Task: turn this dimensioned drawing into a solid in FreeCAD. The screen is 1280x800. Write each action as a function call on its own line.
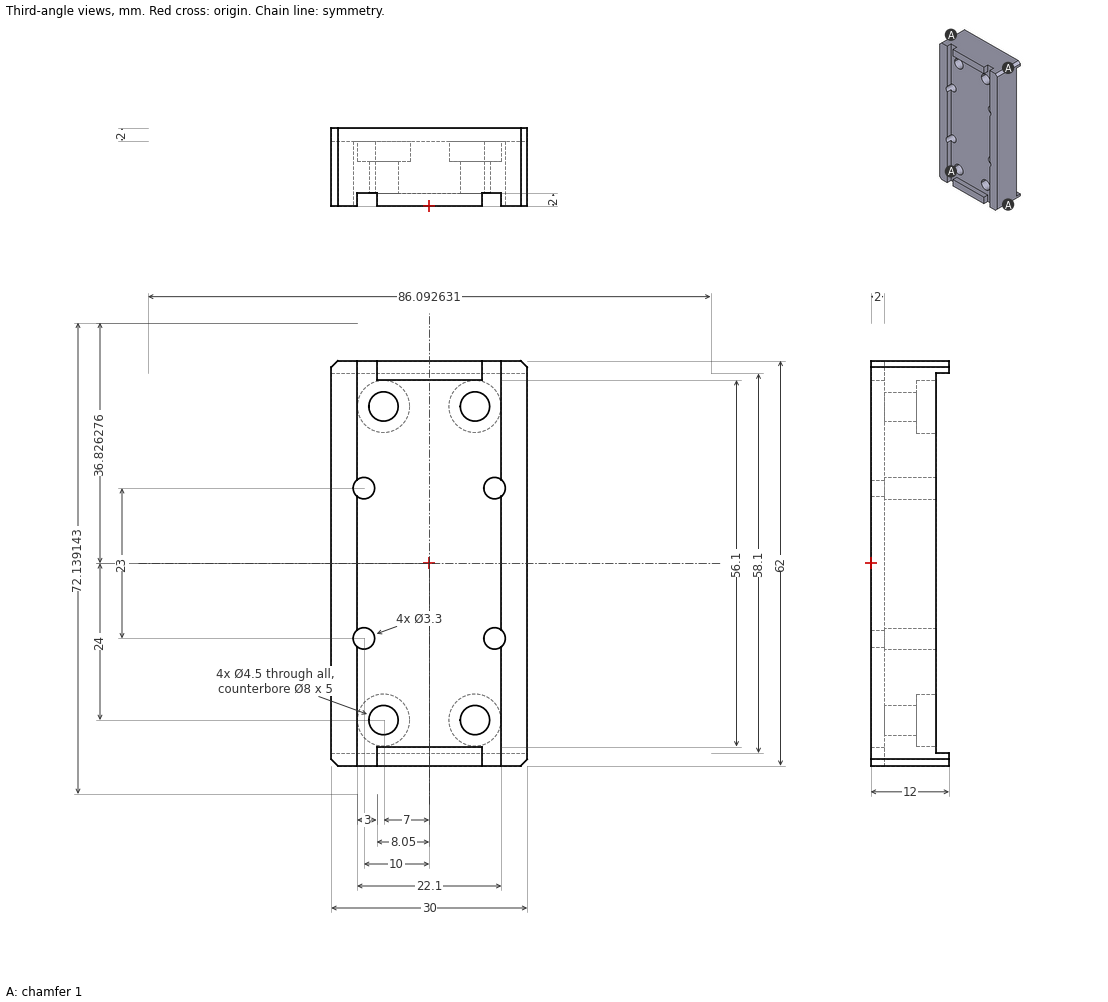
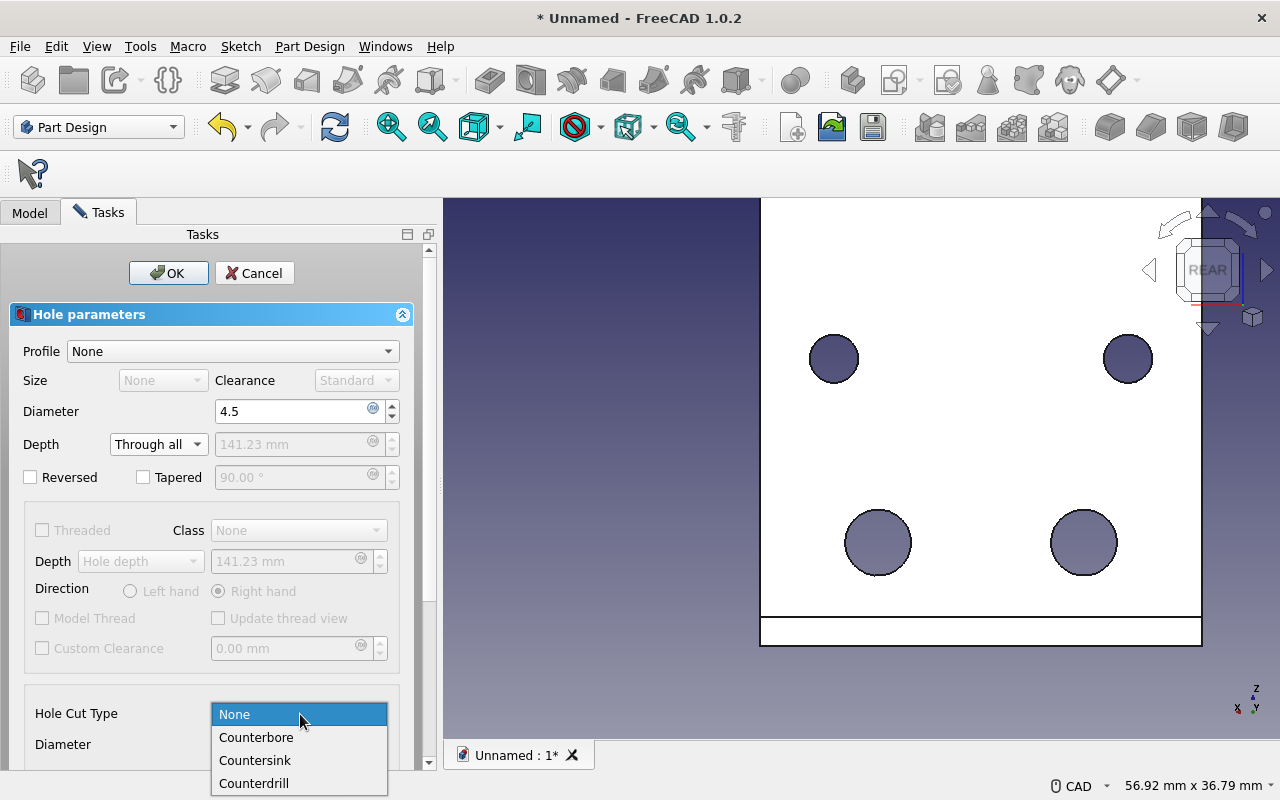
click(298, 738)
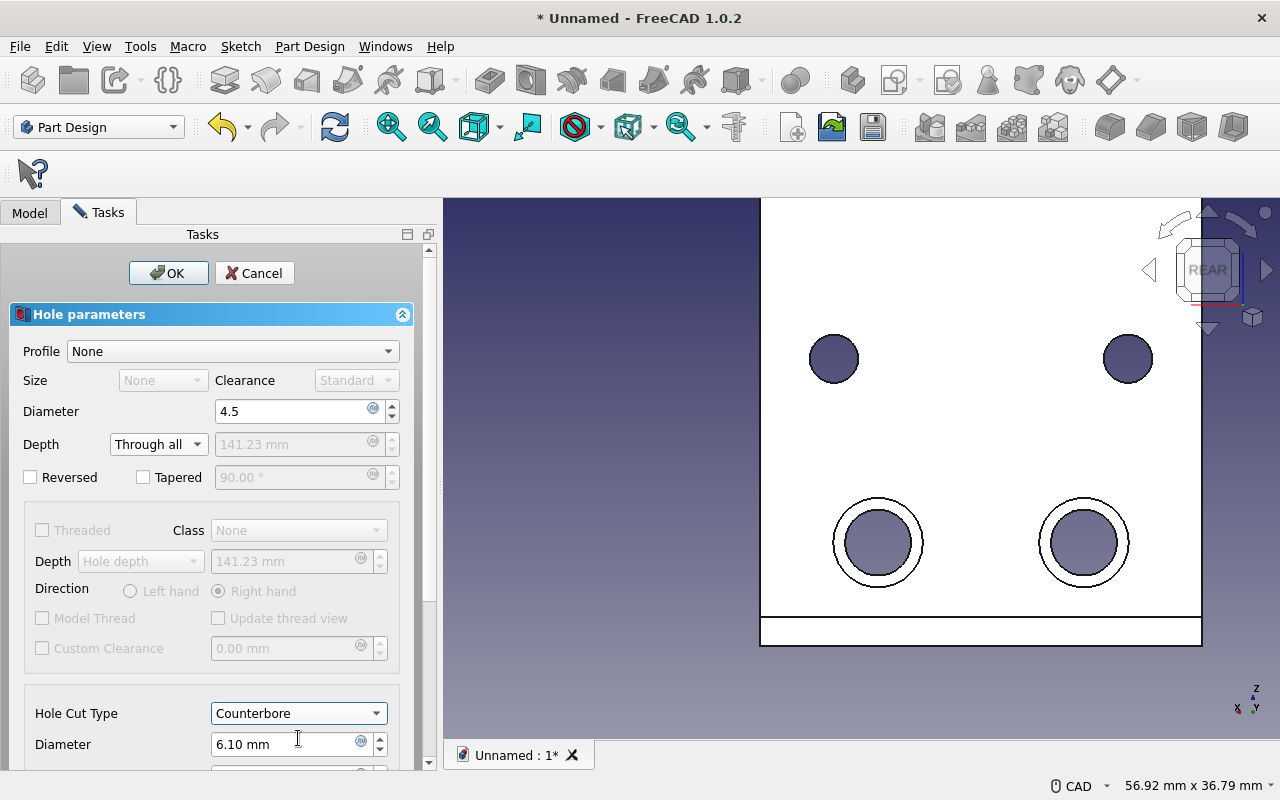
triple_click(292, 744)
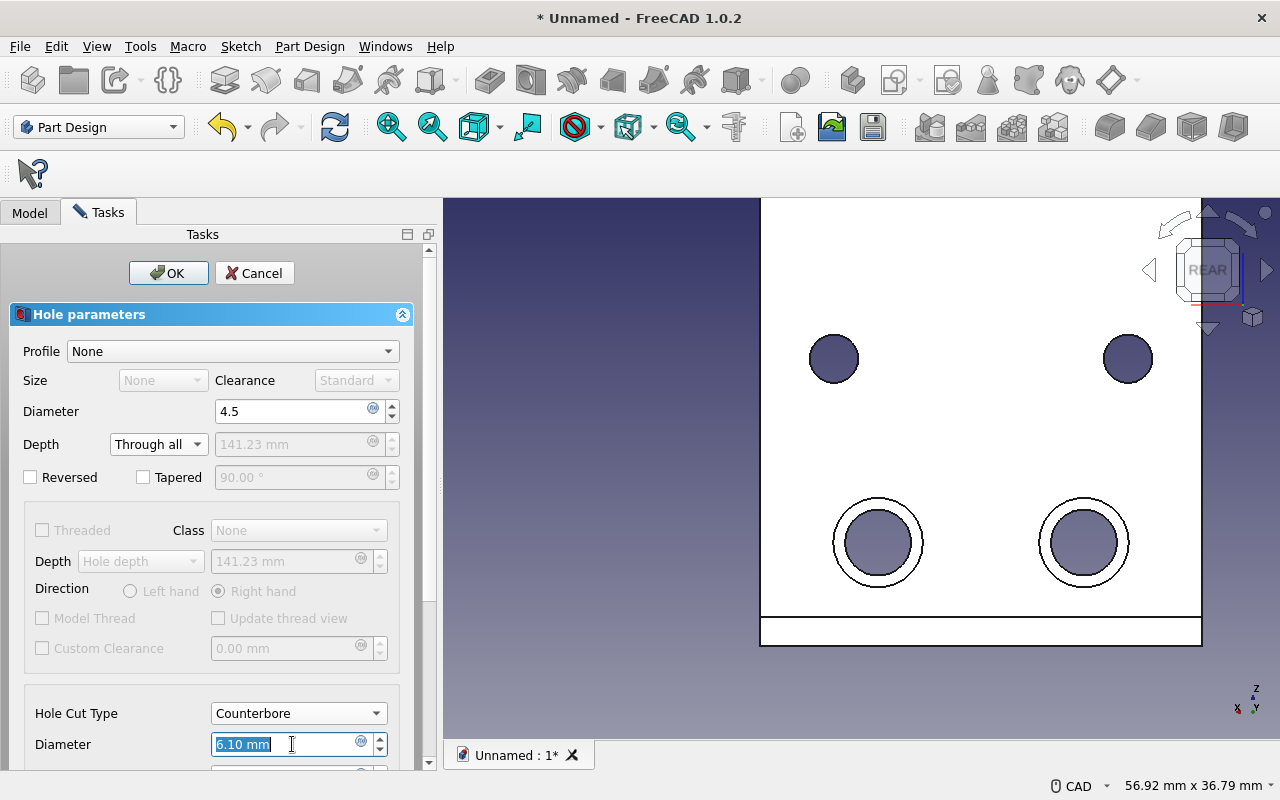
text(8)
key(Tab)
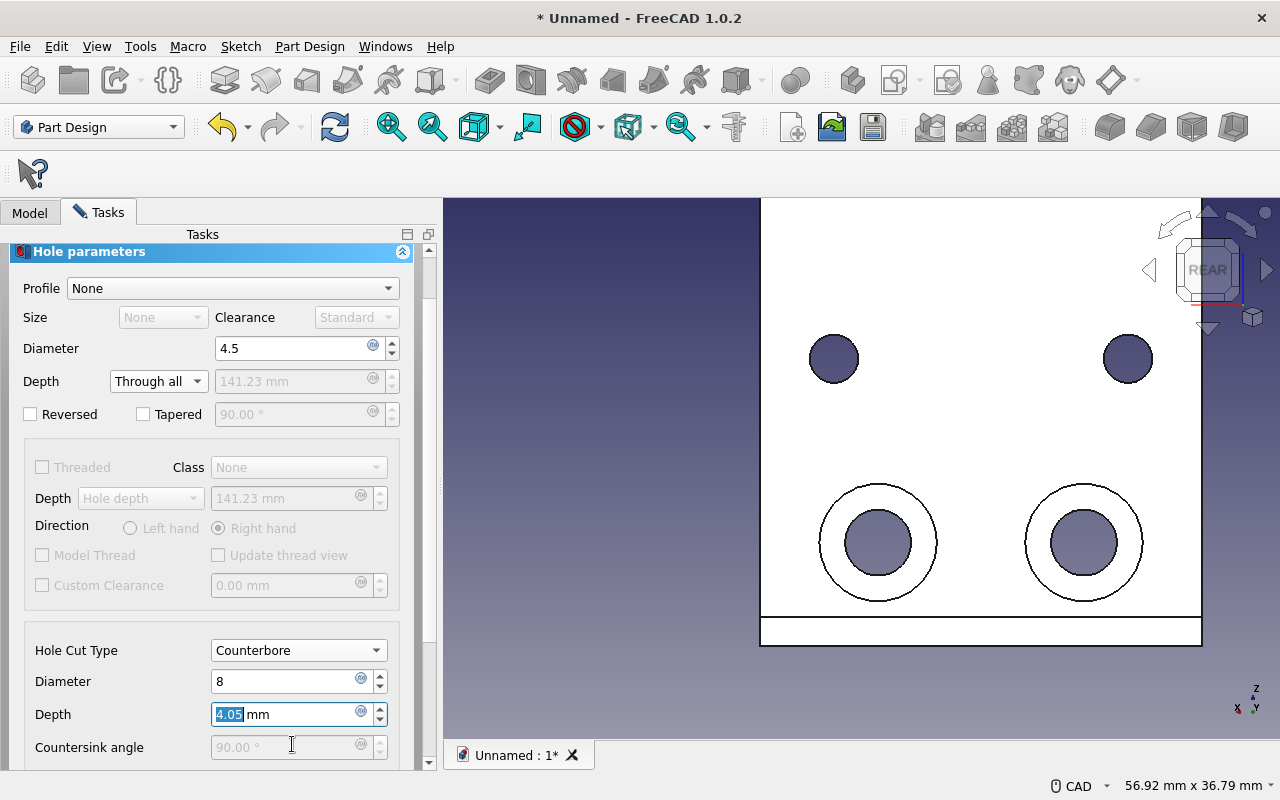
text(5)
key(Tab)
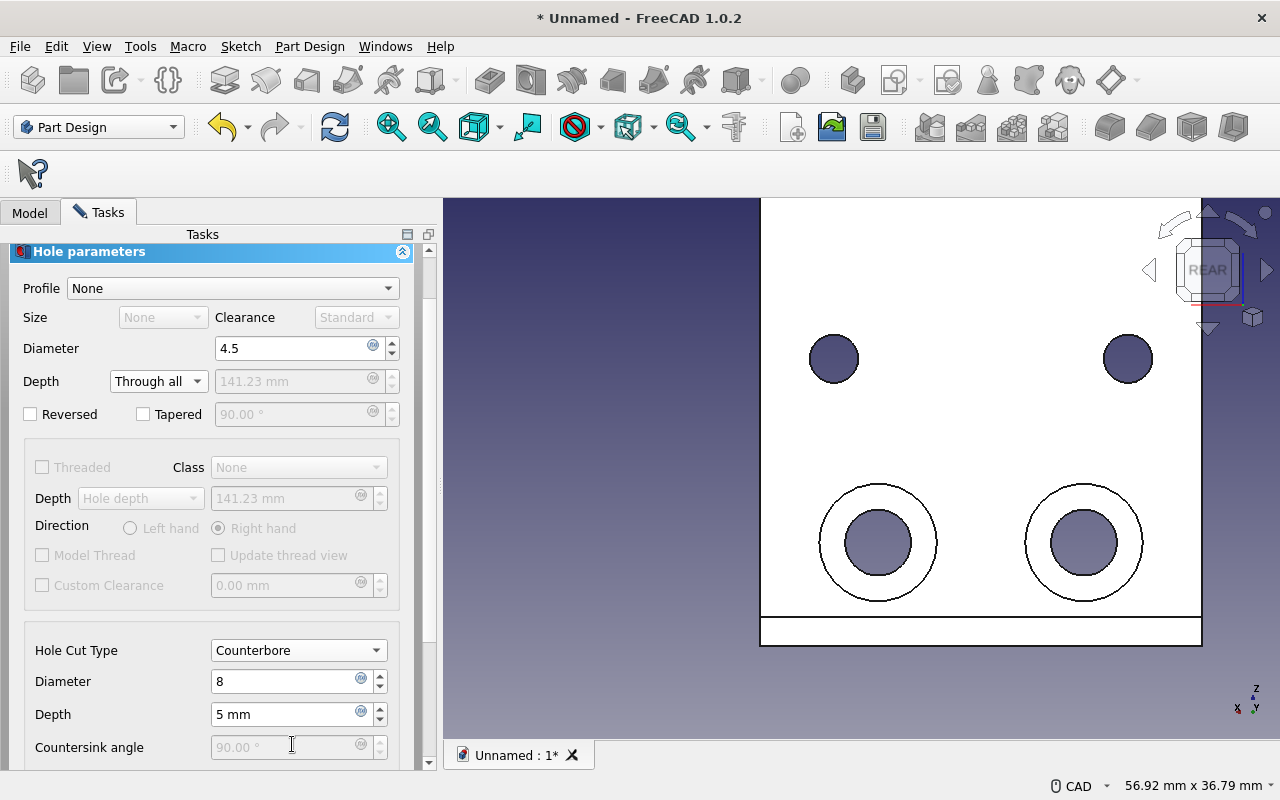
scroll(429, 507, up, 2)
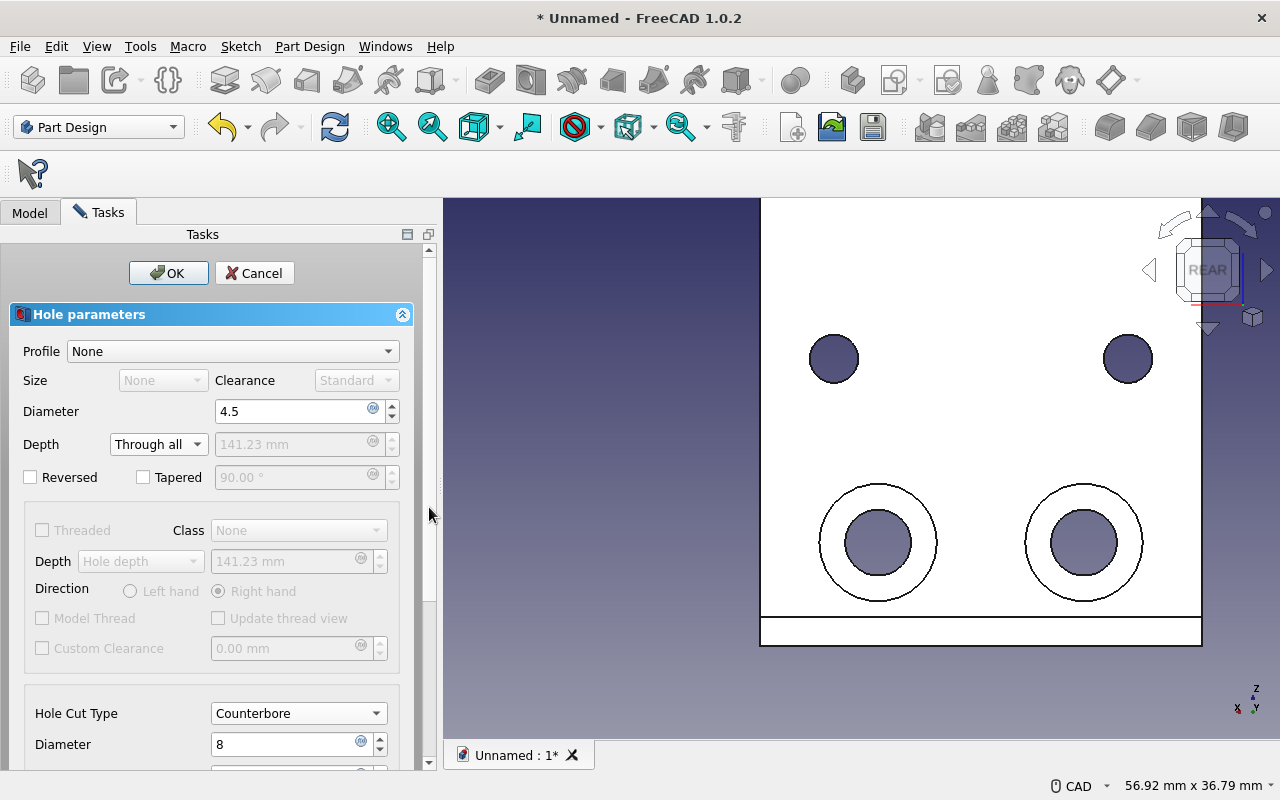
click(169, 273)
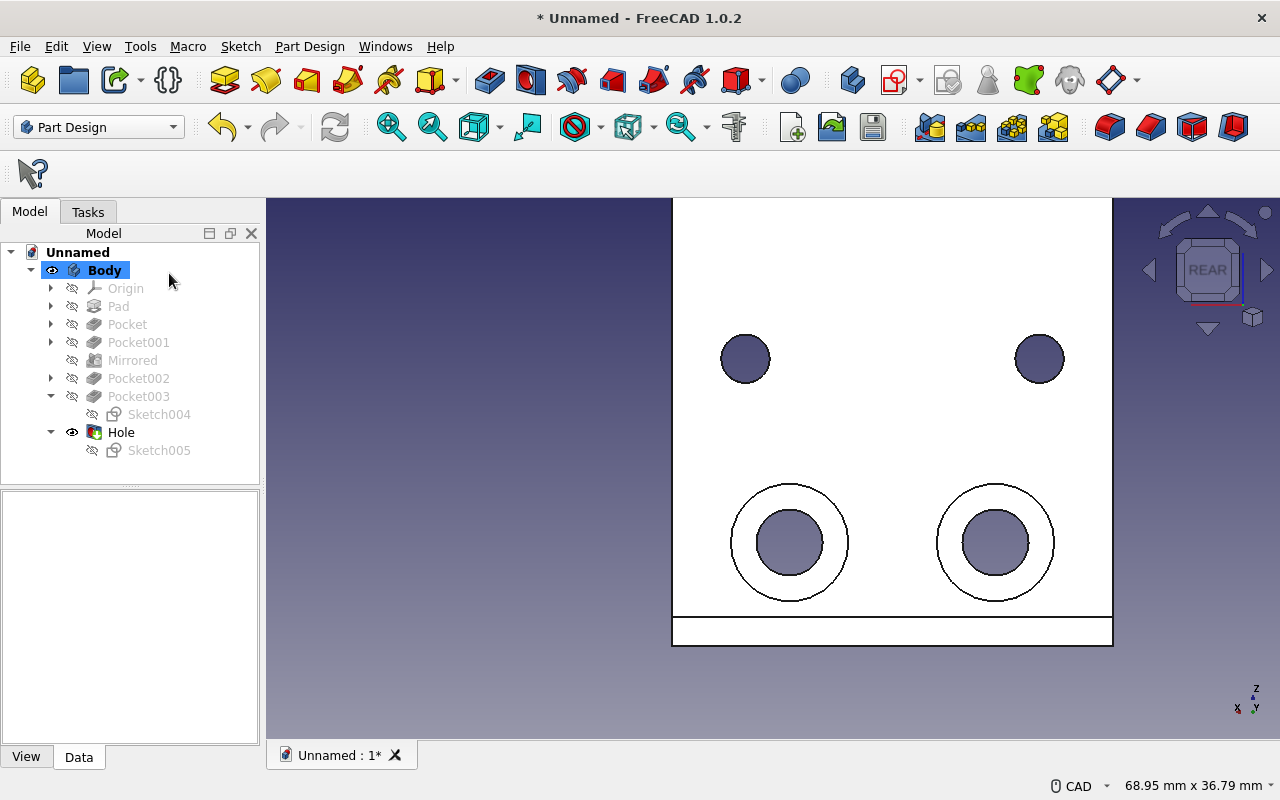
click(392, 128)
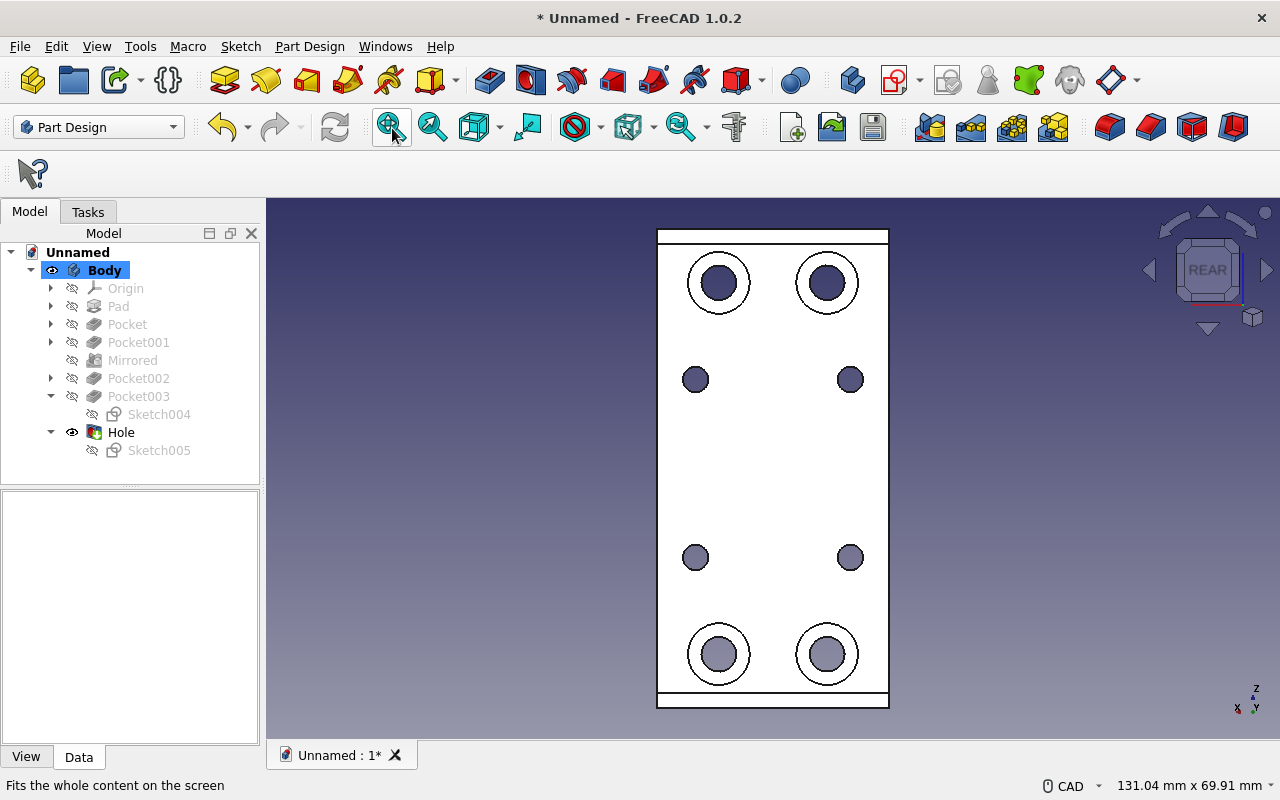
key(0)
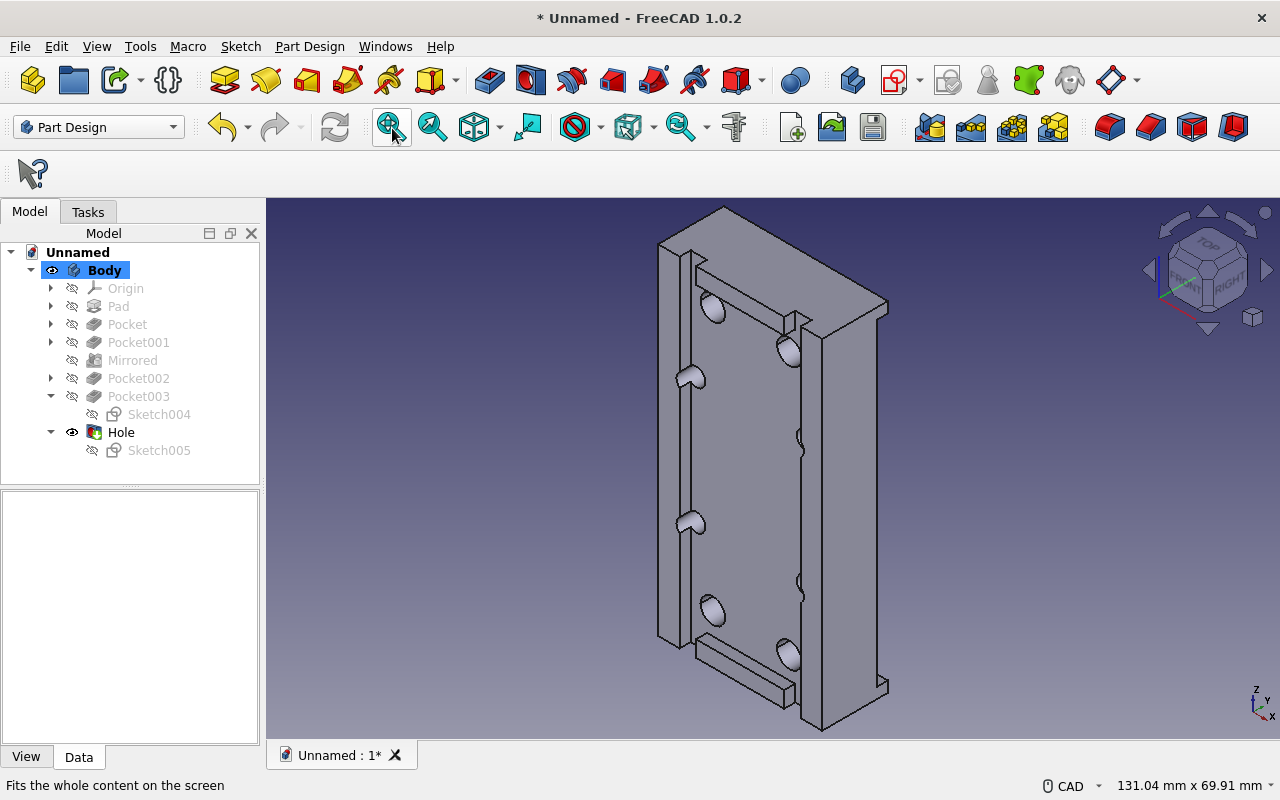
click(855, 319)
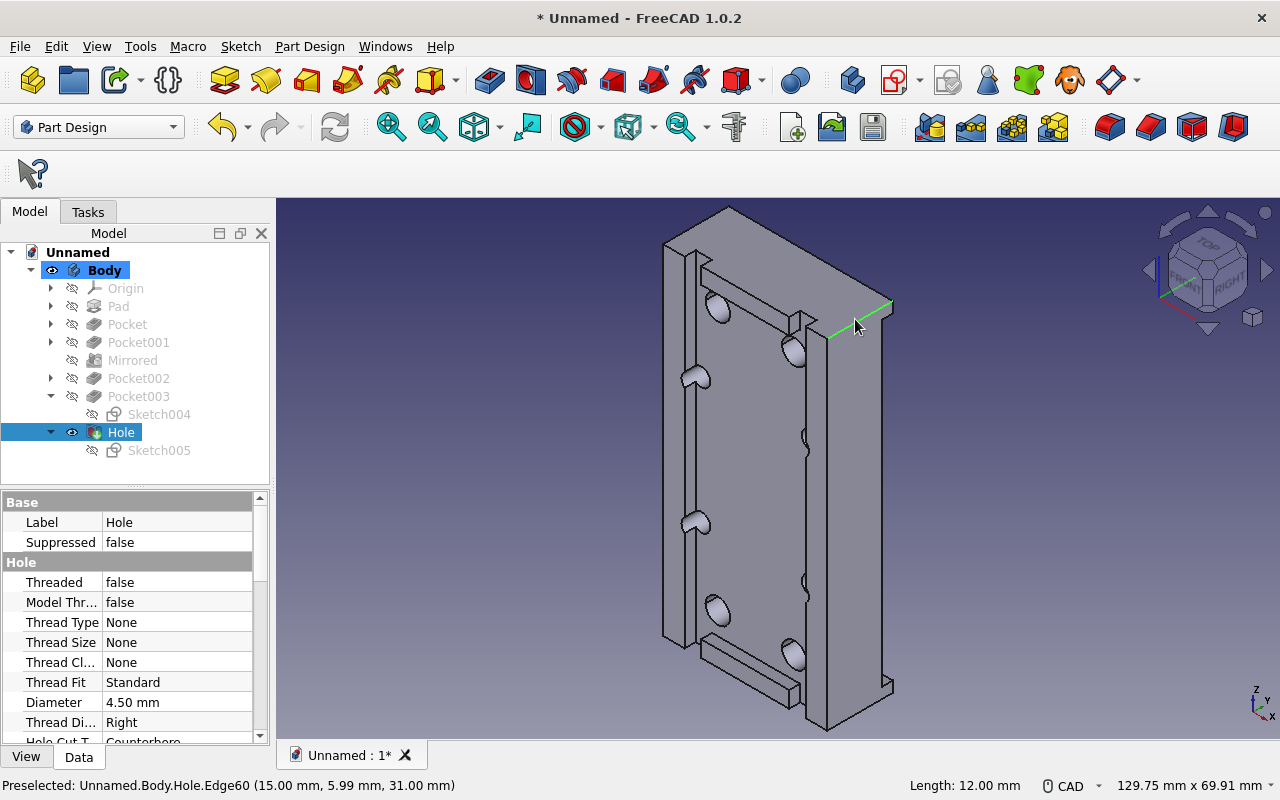
key(2)